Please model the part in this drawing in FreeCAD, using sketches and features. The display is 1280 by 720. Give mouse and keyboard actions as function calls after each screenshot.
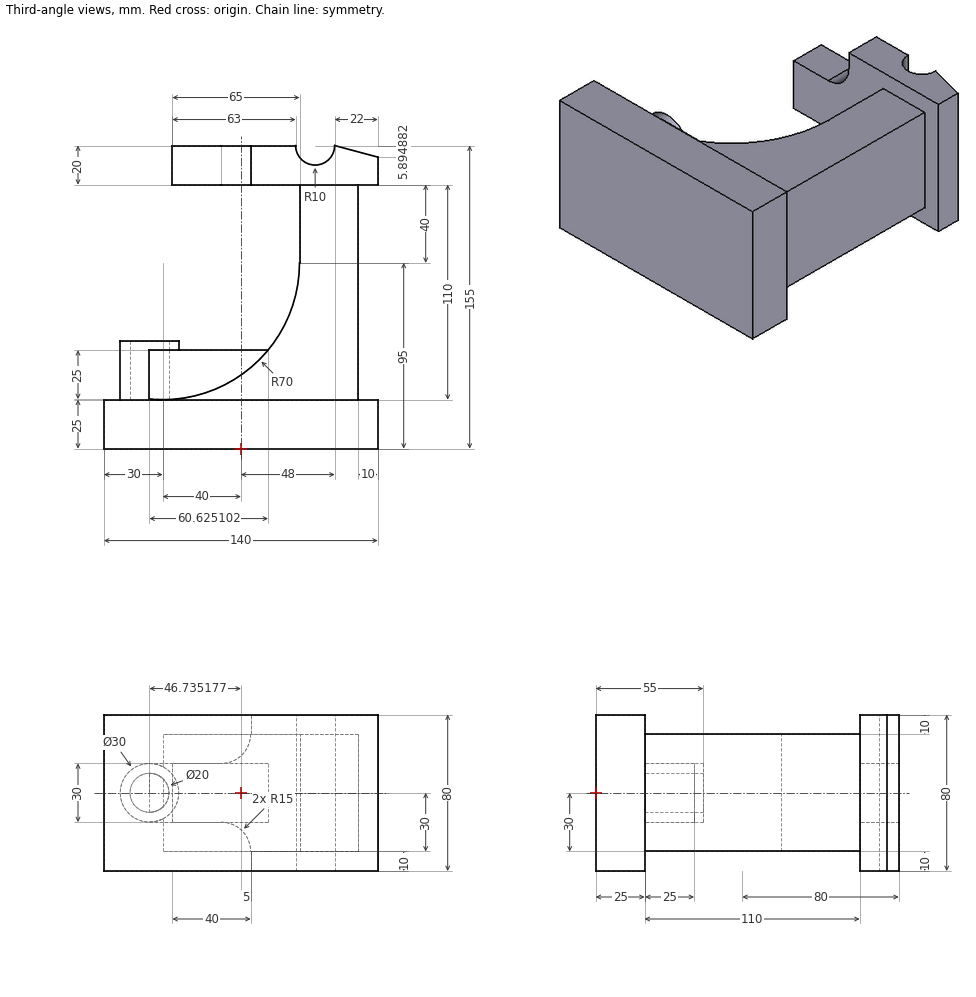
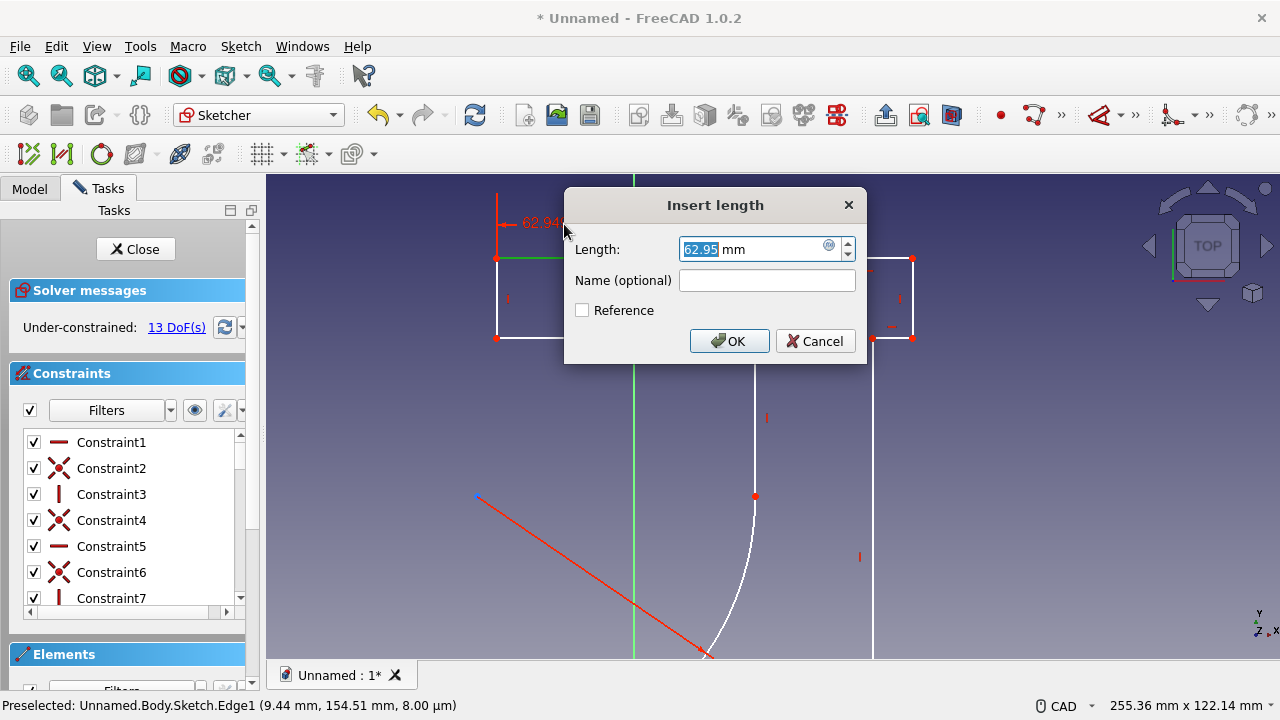
text(63)
key(Return)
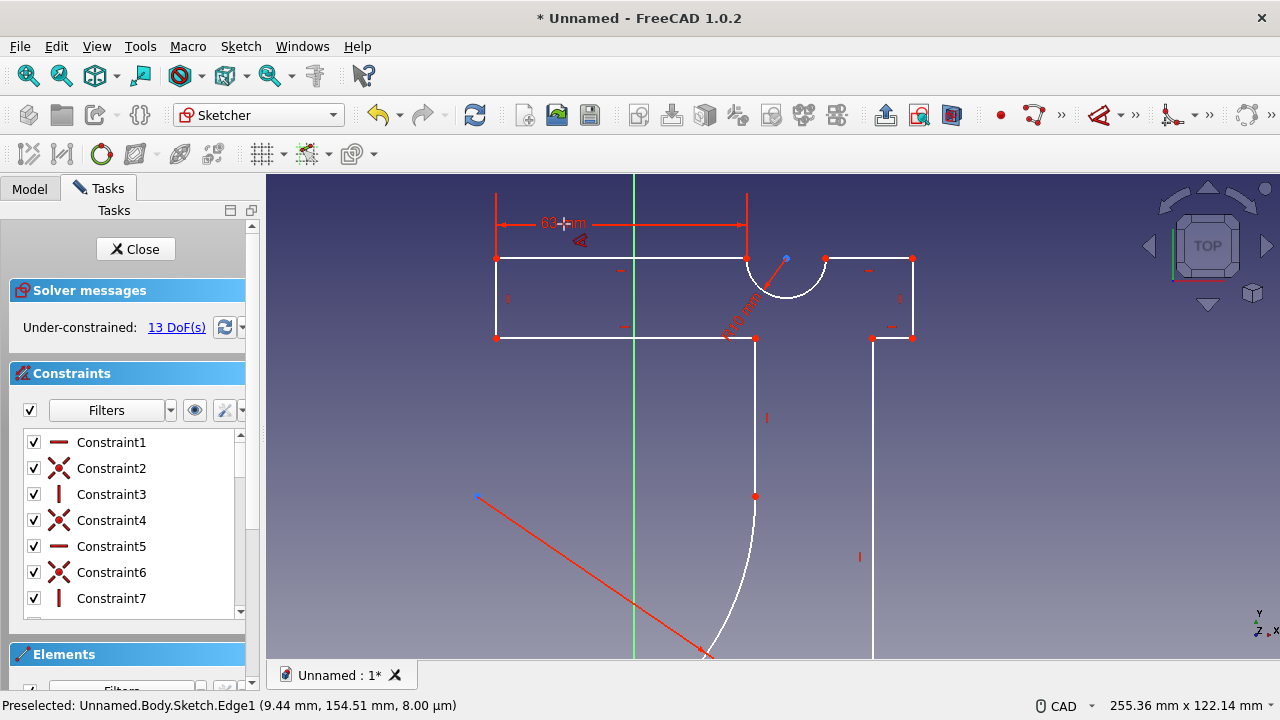
click(496, 282)
click(462, 298)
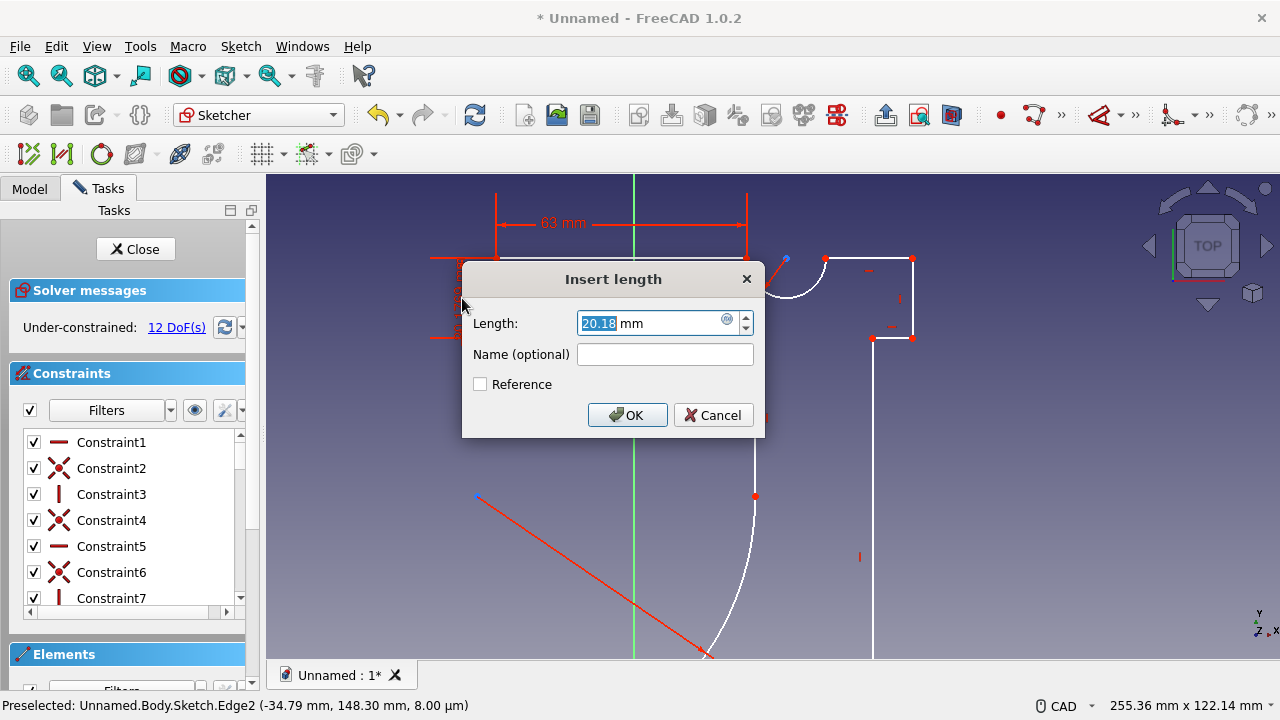
text(20)
key(Return)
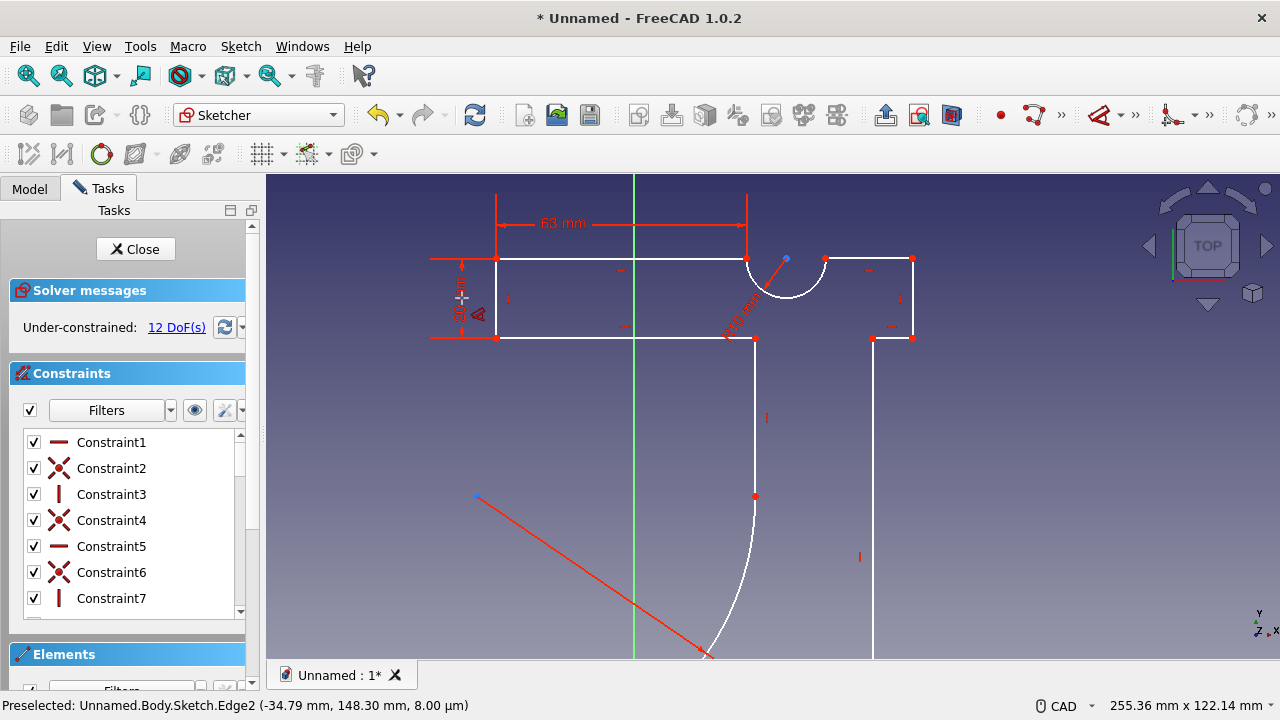
click(574, 338)
click(566, 304)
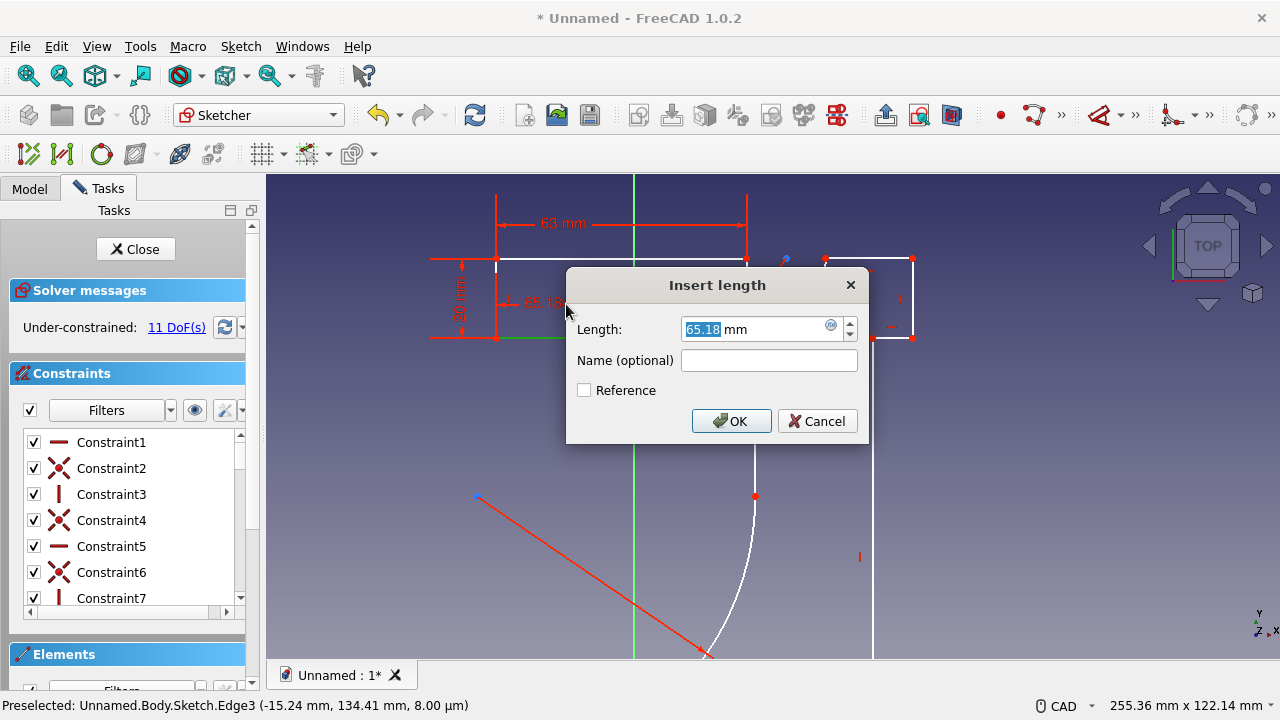
text(65)
key(Return)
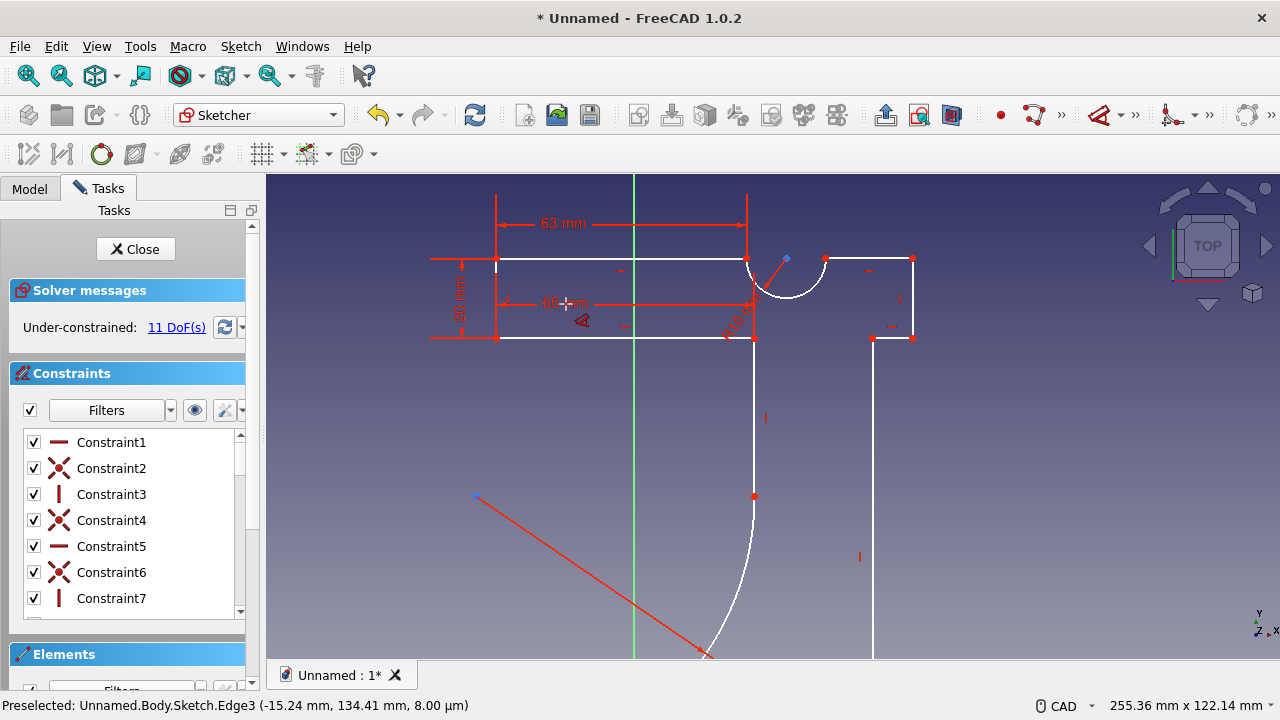
click(754, 386)
click(788, 417)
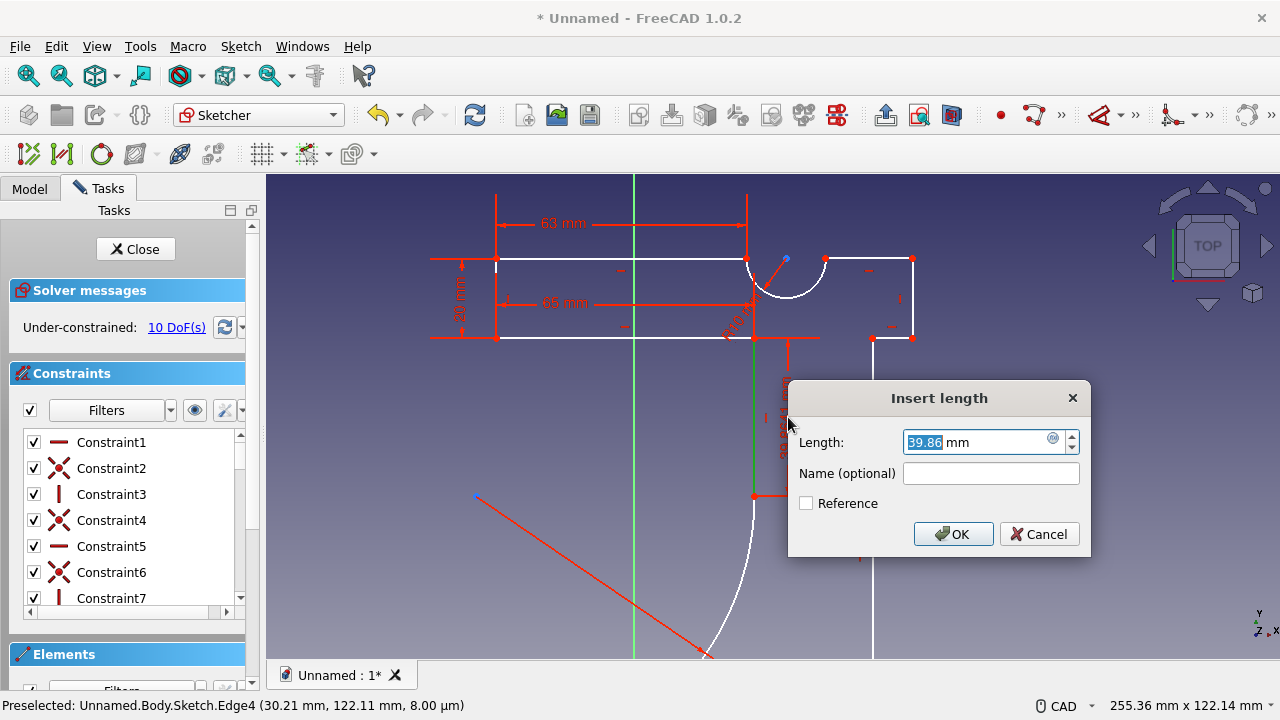
text(40)
key(Return)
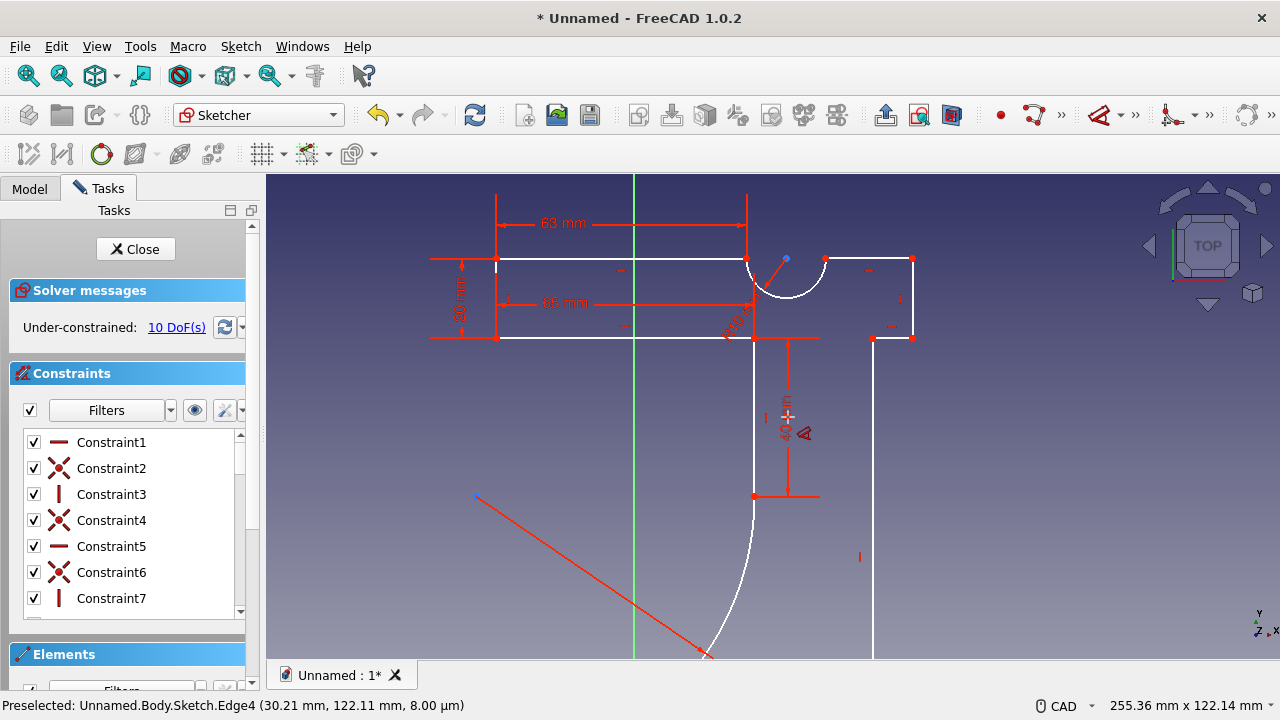
scroll(762, 296, down, 4)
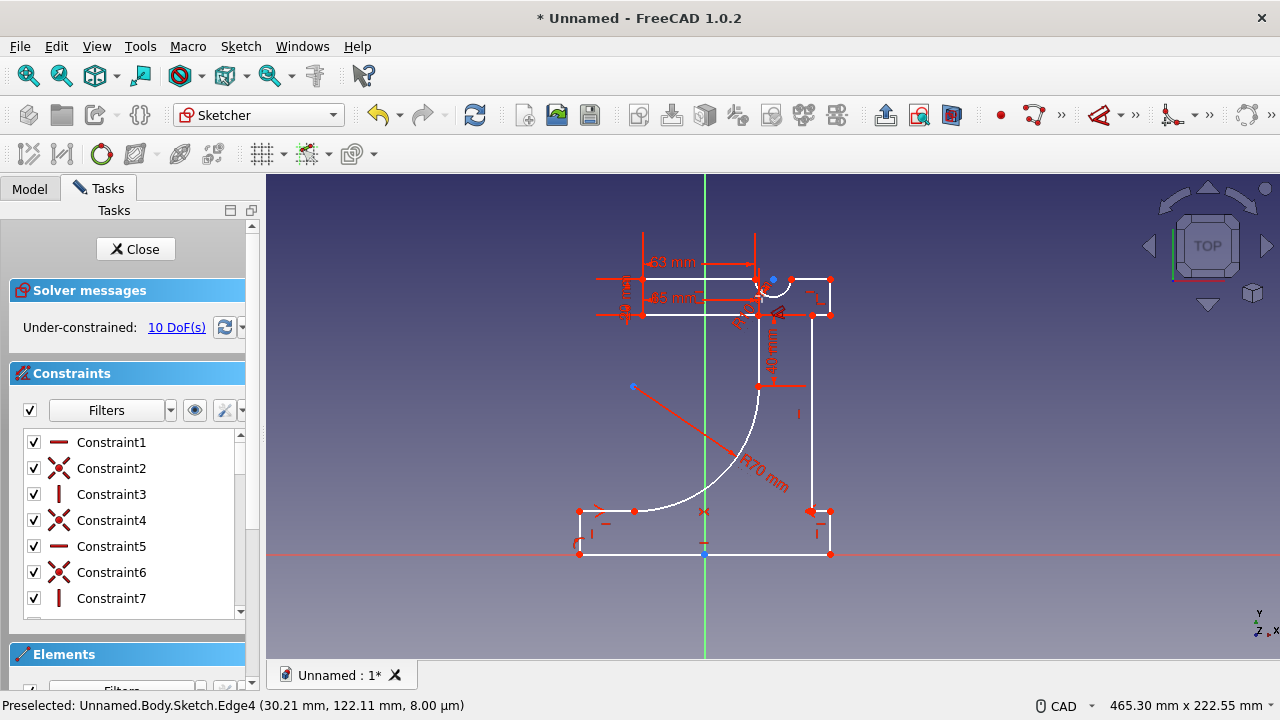
click(618, 511)
click(607, 477)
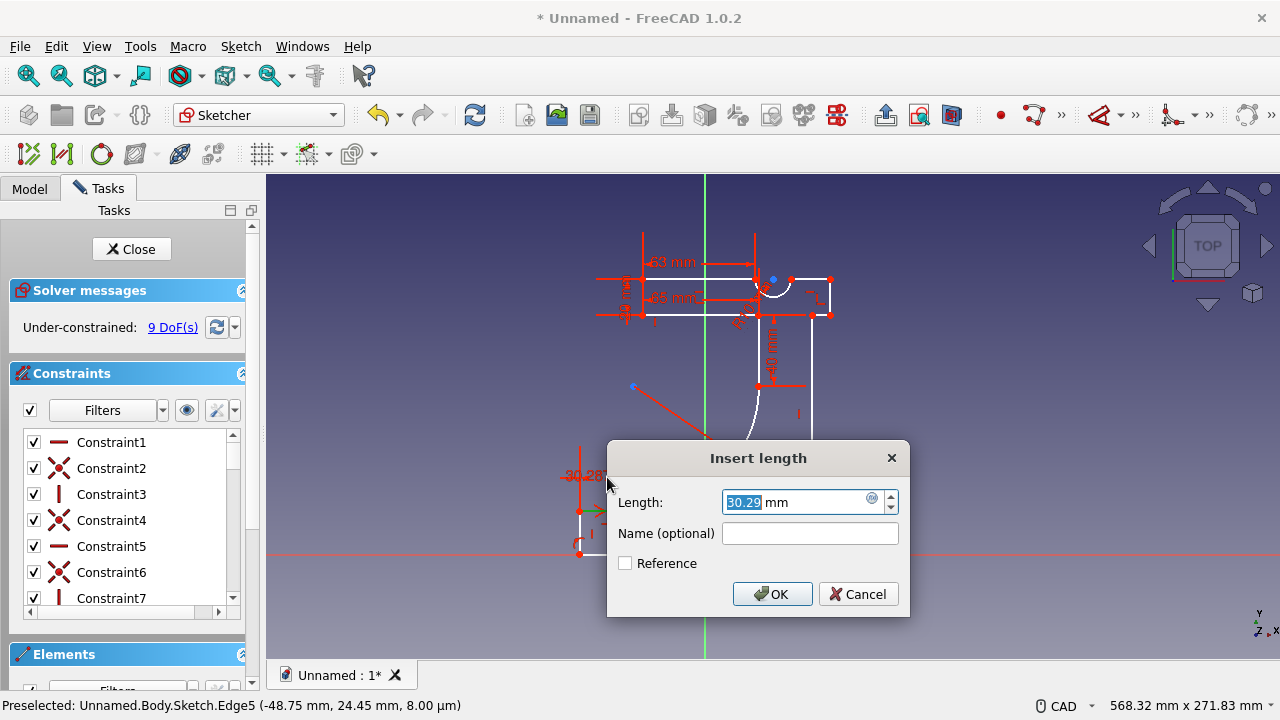
text(30)
key(Return)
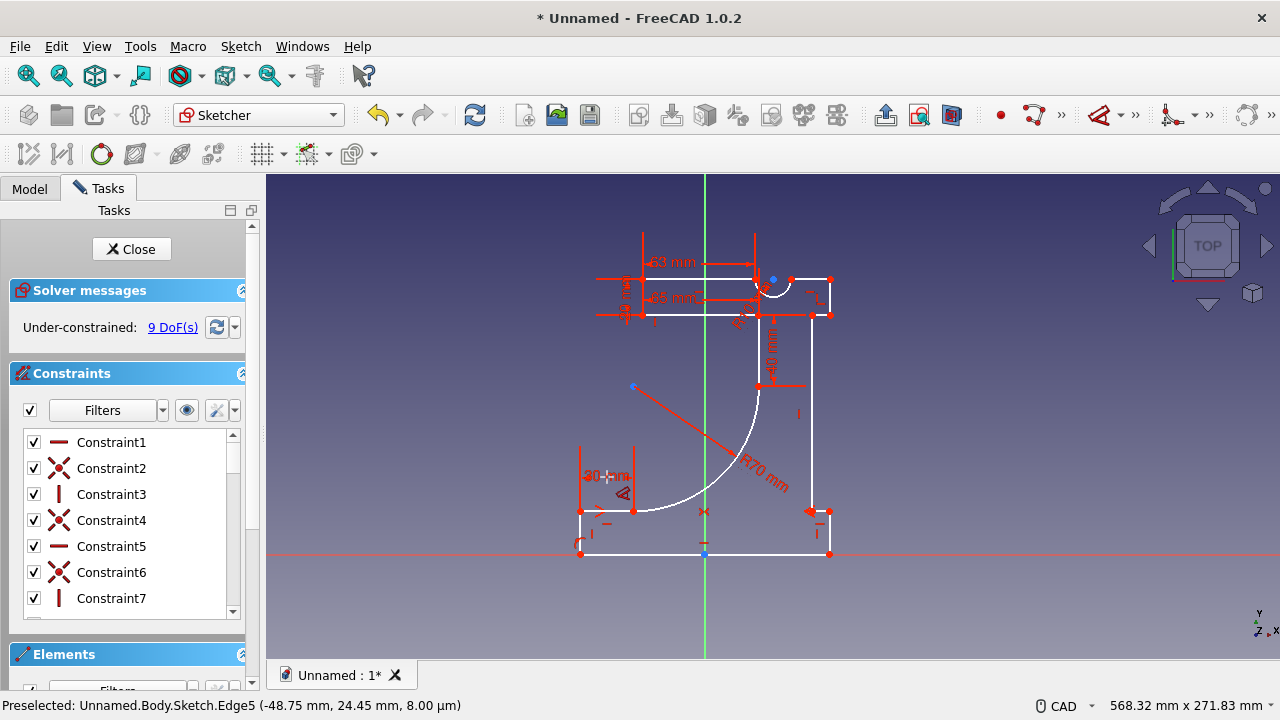
click(580, 524)
click(546, 533)